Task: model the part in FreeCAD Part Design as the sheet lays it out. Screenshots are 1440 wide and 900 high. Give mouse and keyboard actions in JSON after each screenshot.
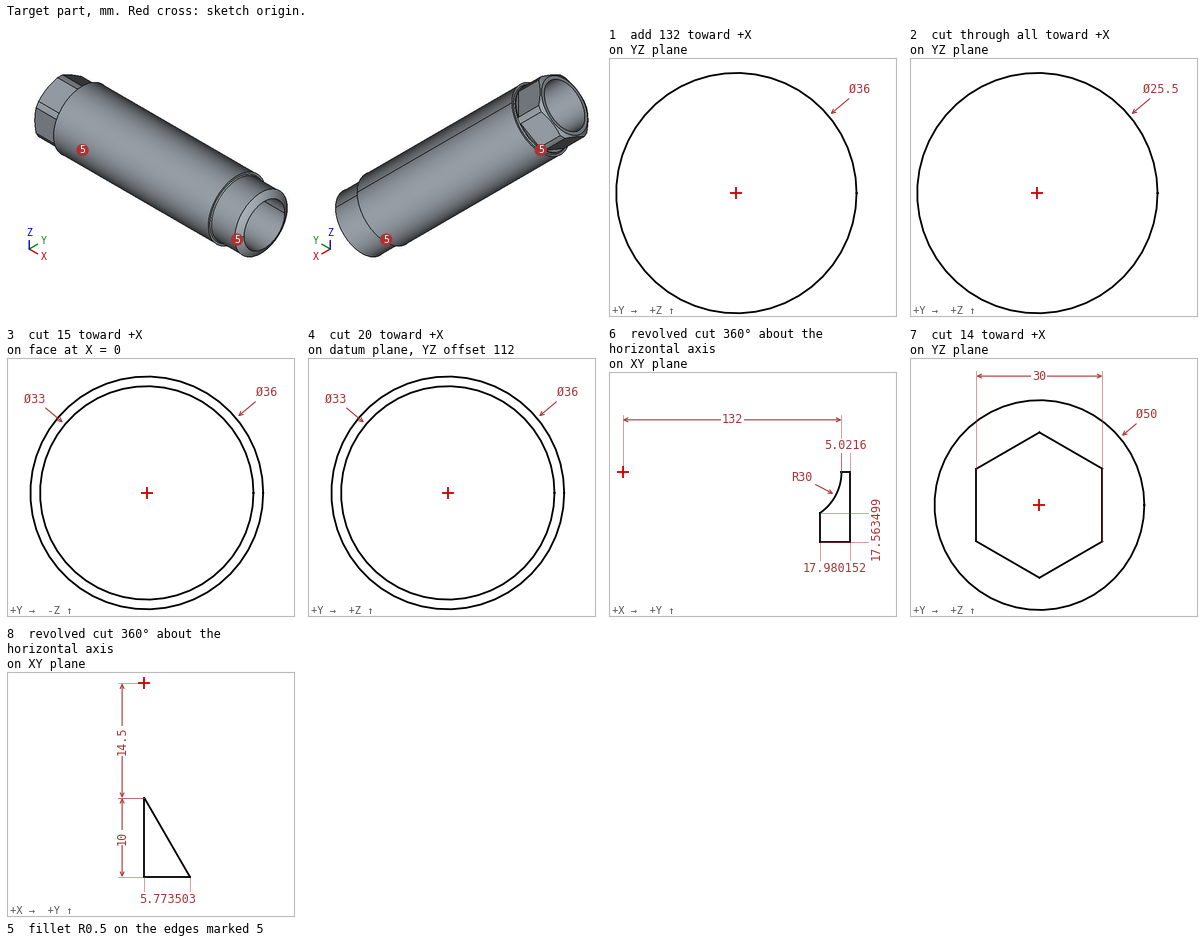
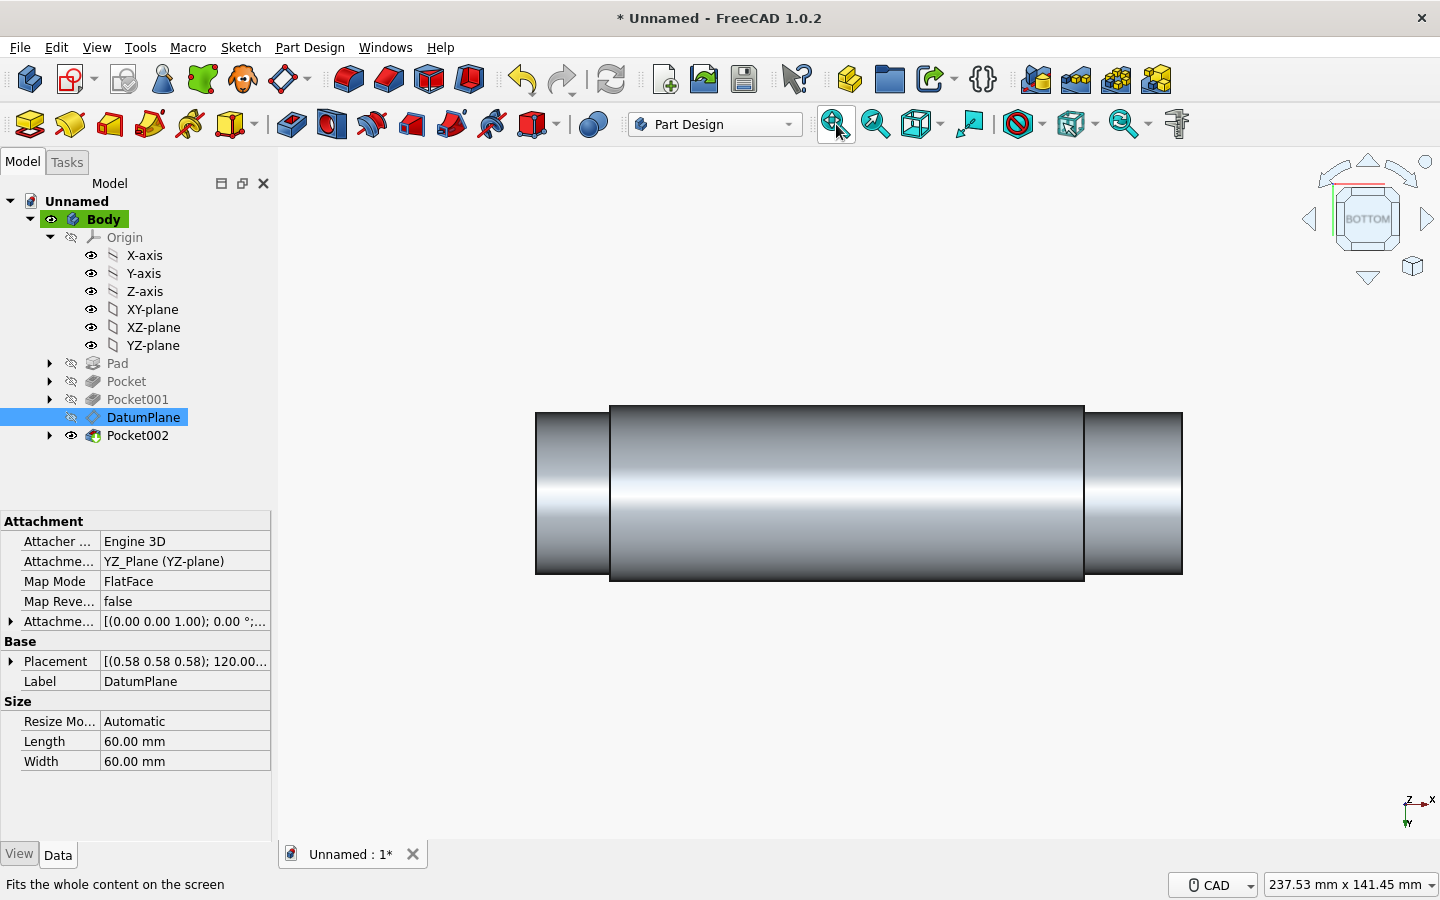
{"action": "key", "text": "4"}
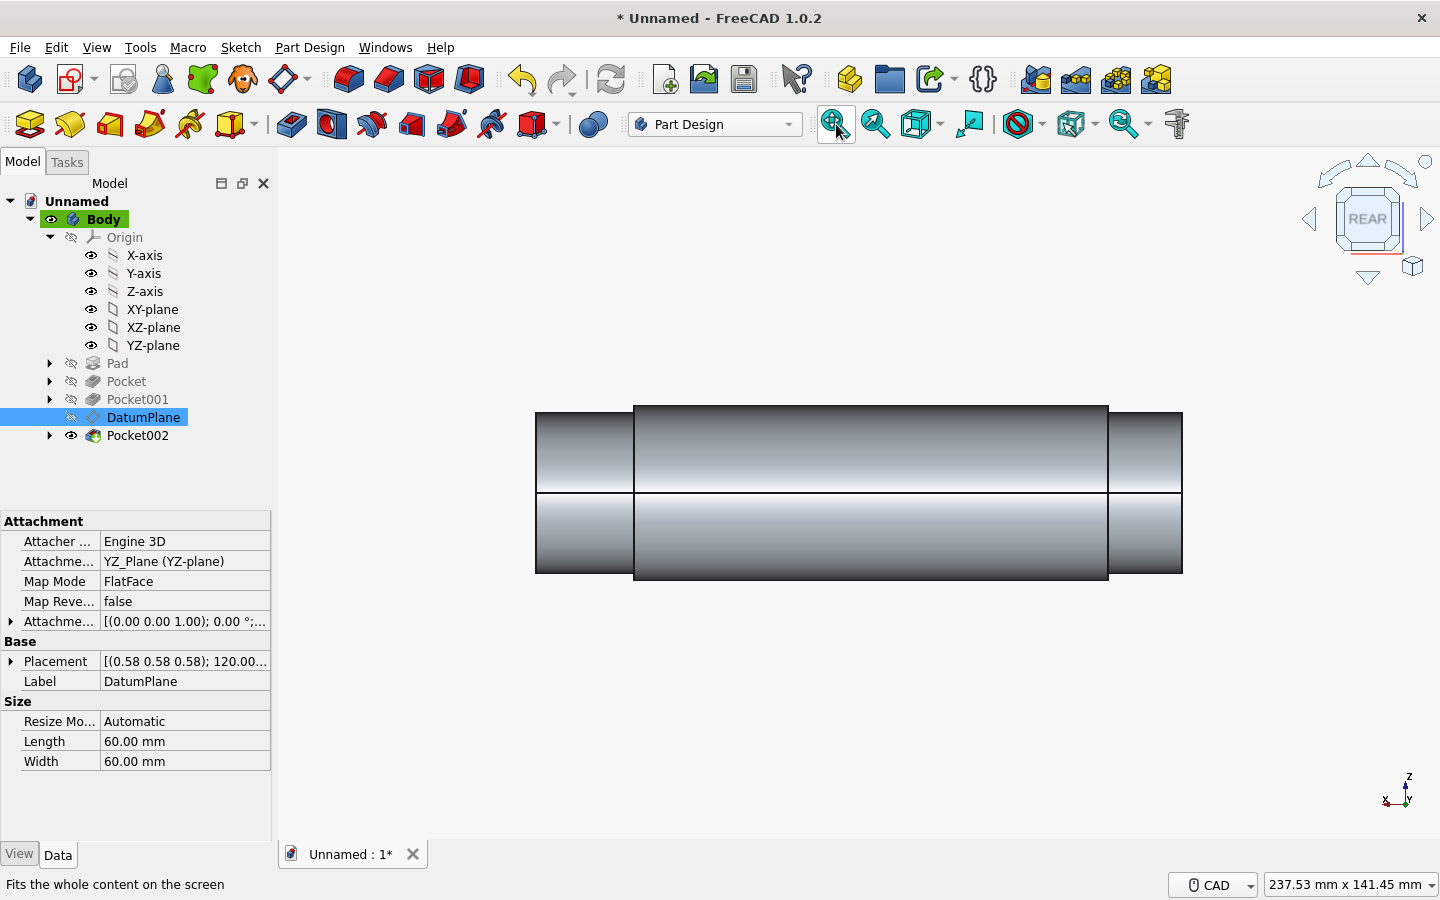
{"action": "key", "text": "6"}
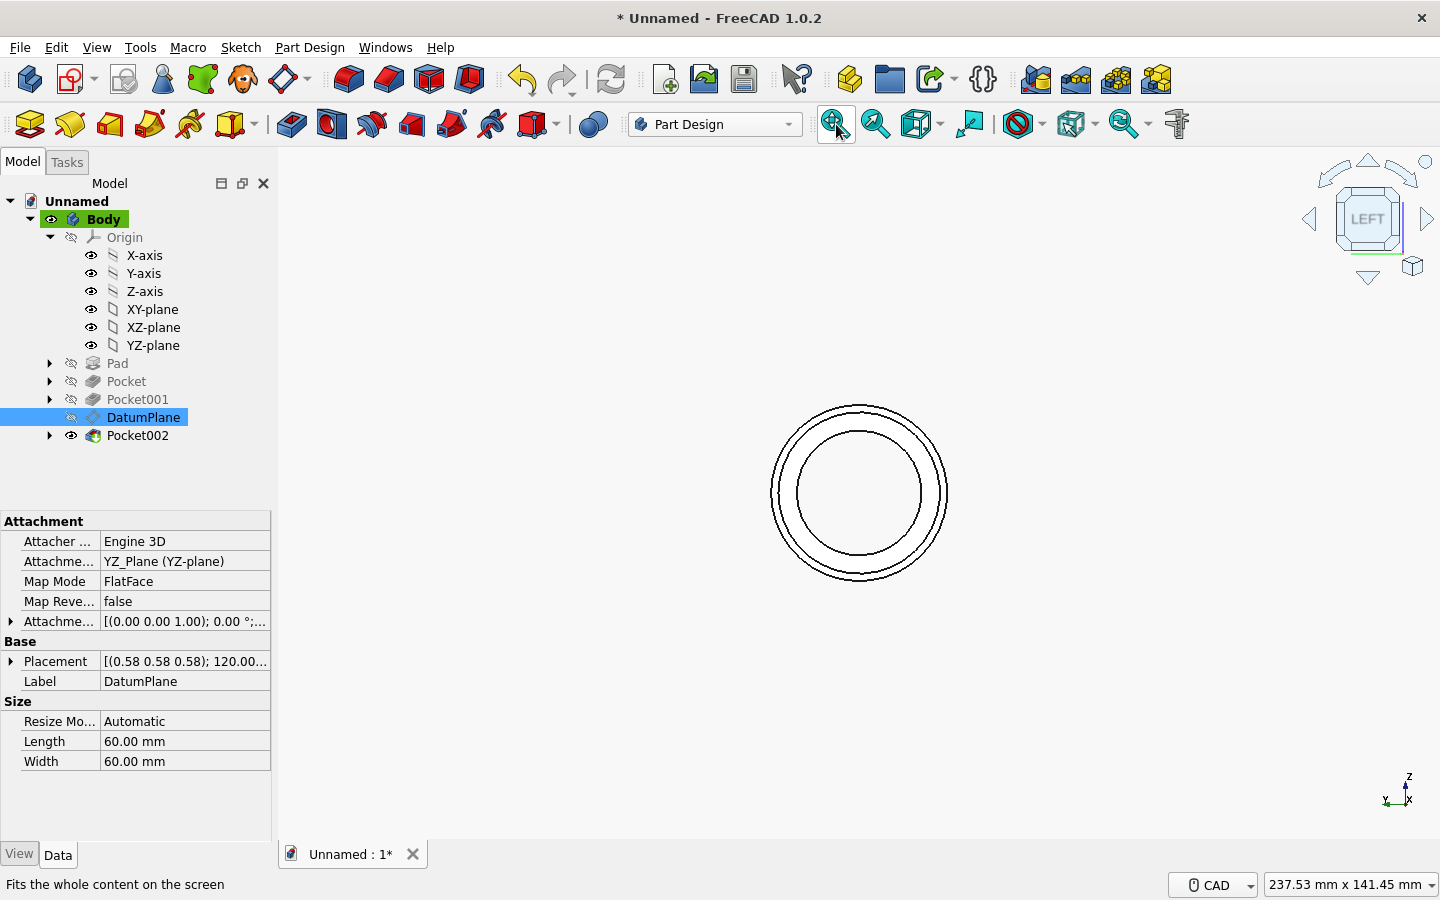
{"action": "left_click", "coordinate": [836, 124]}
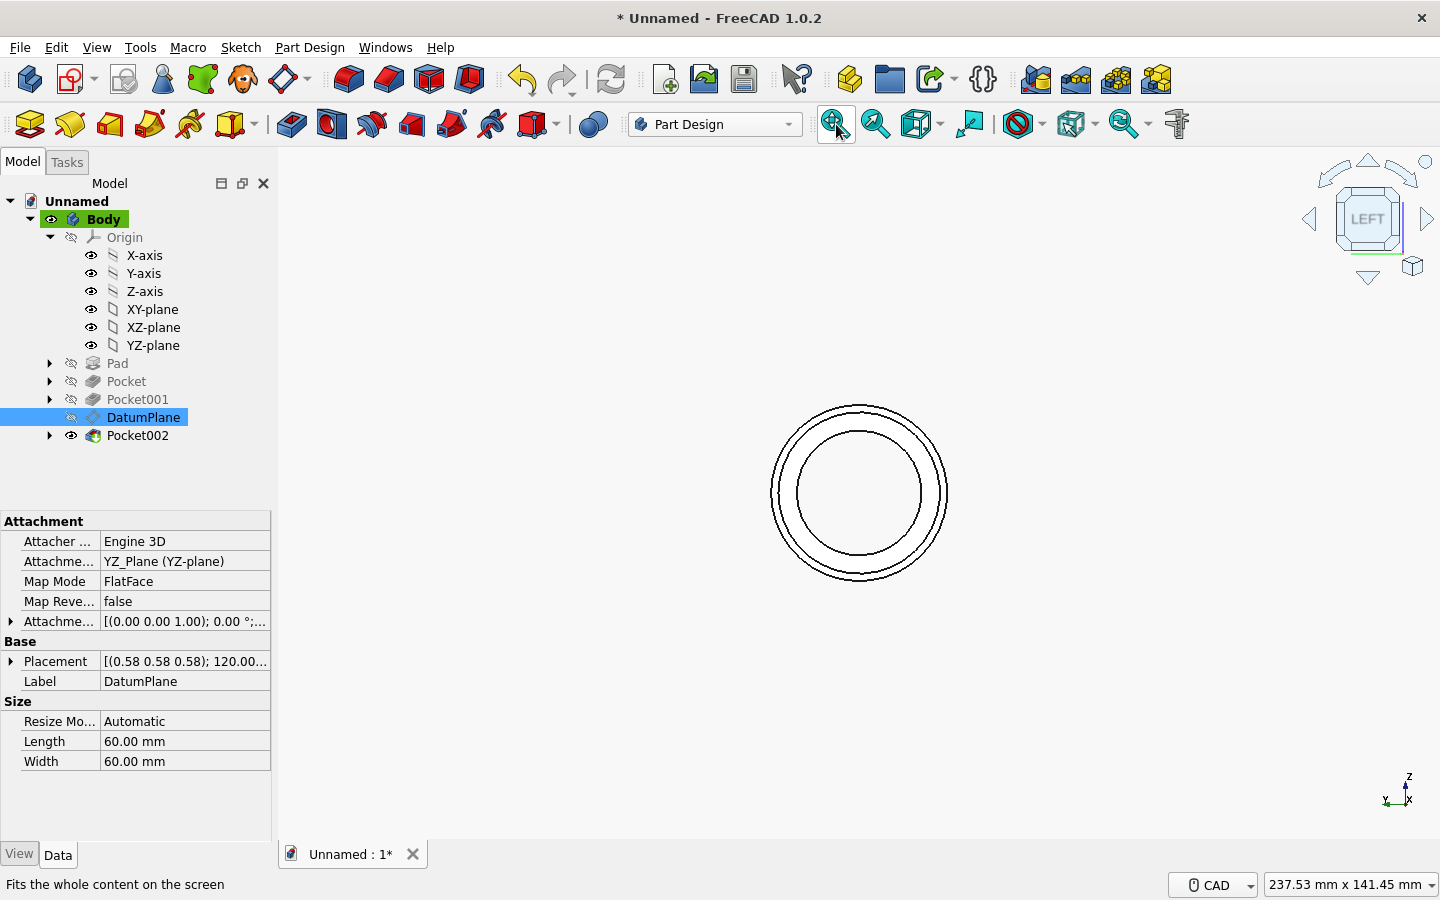
{"action": "key", "text": "v 3"}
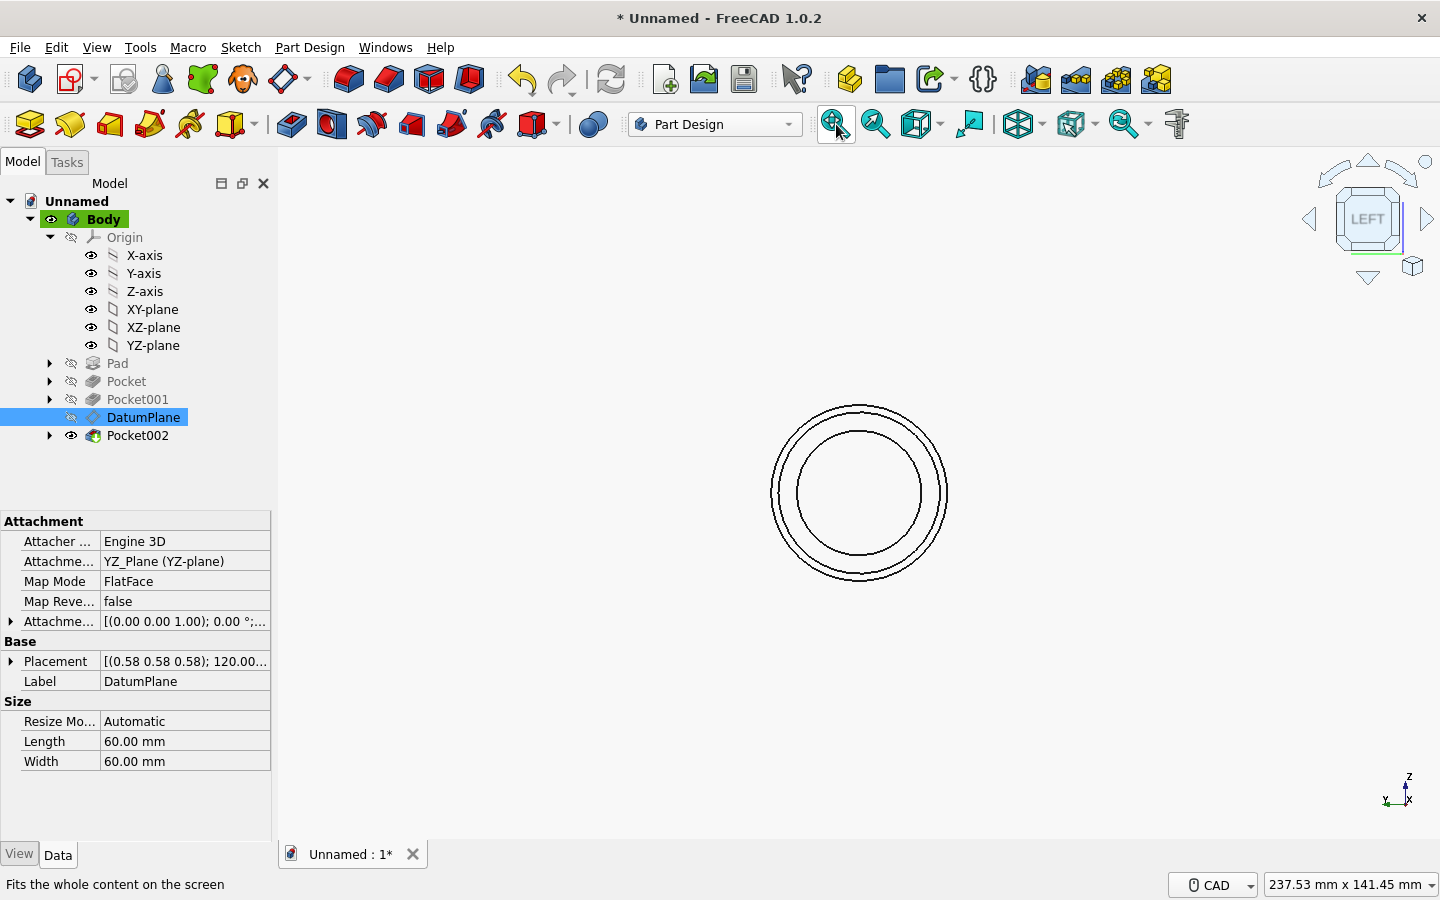
{"action": "key", "text": "0"}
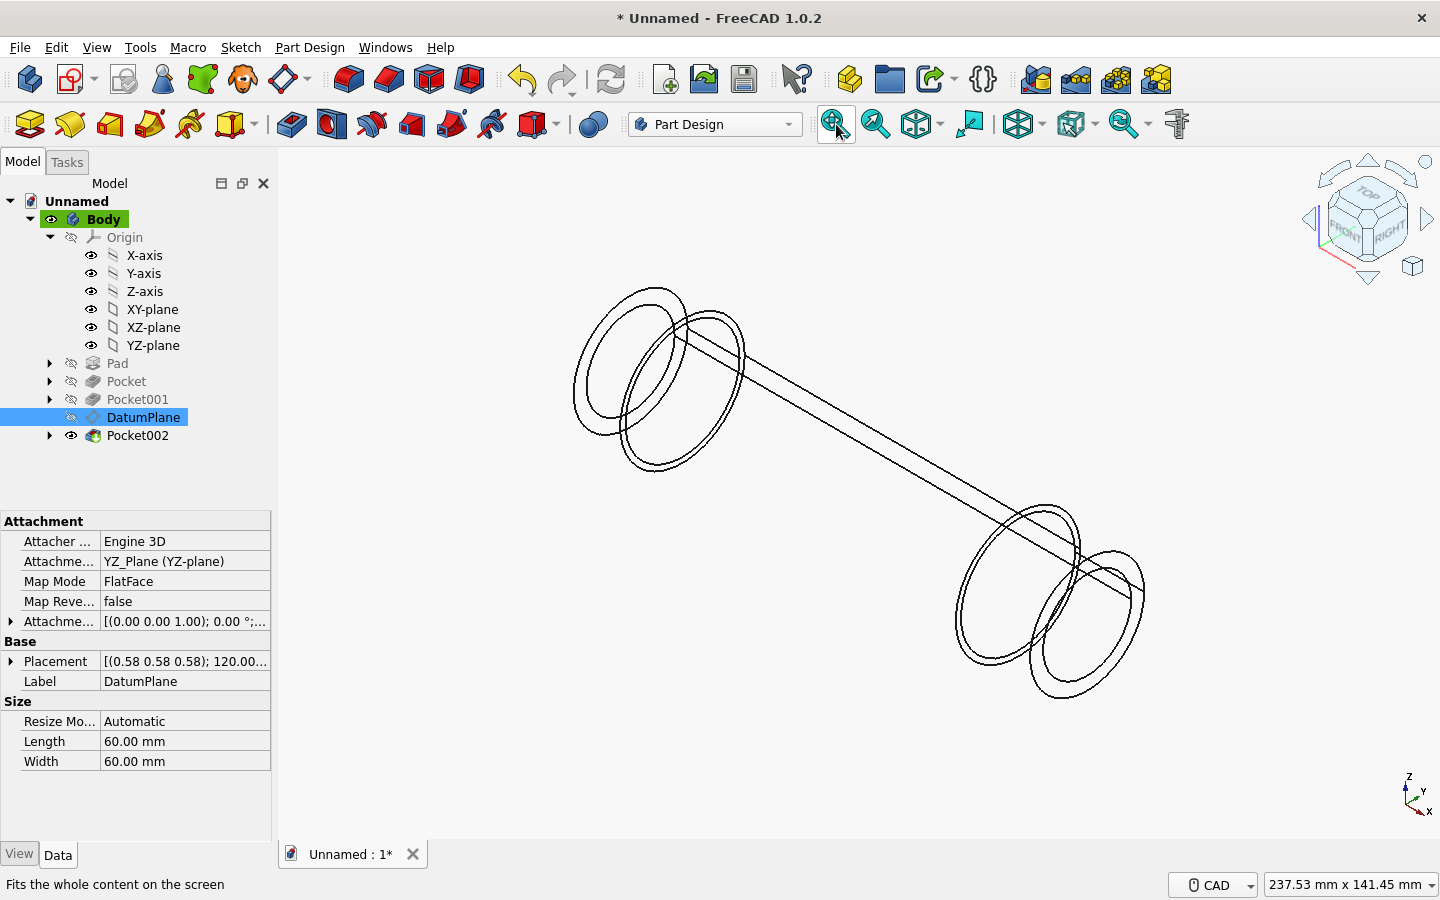
{"action": "left_click", "coordinate": [636, 456]}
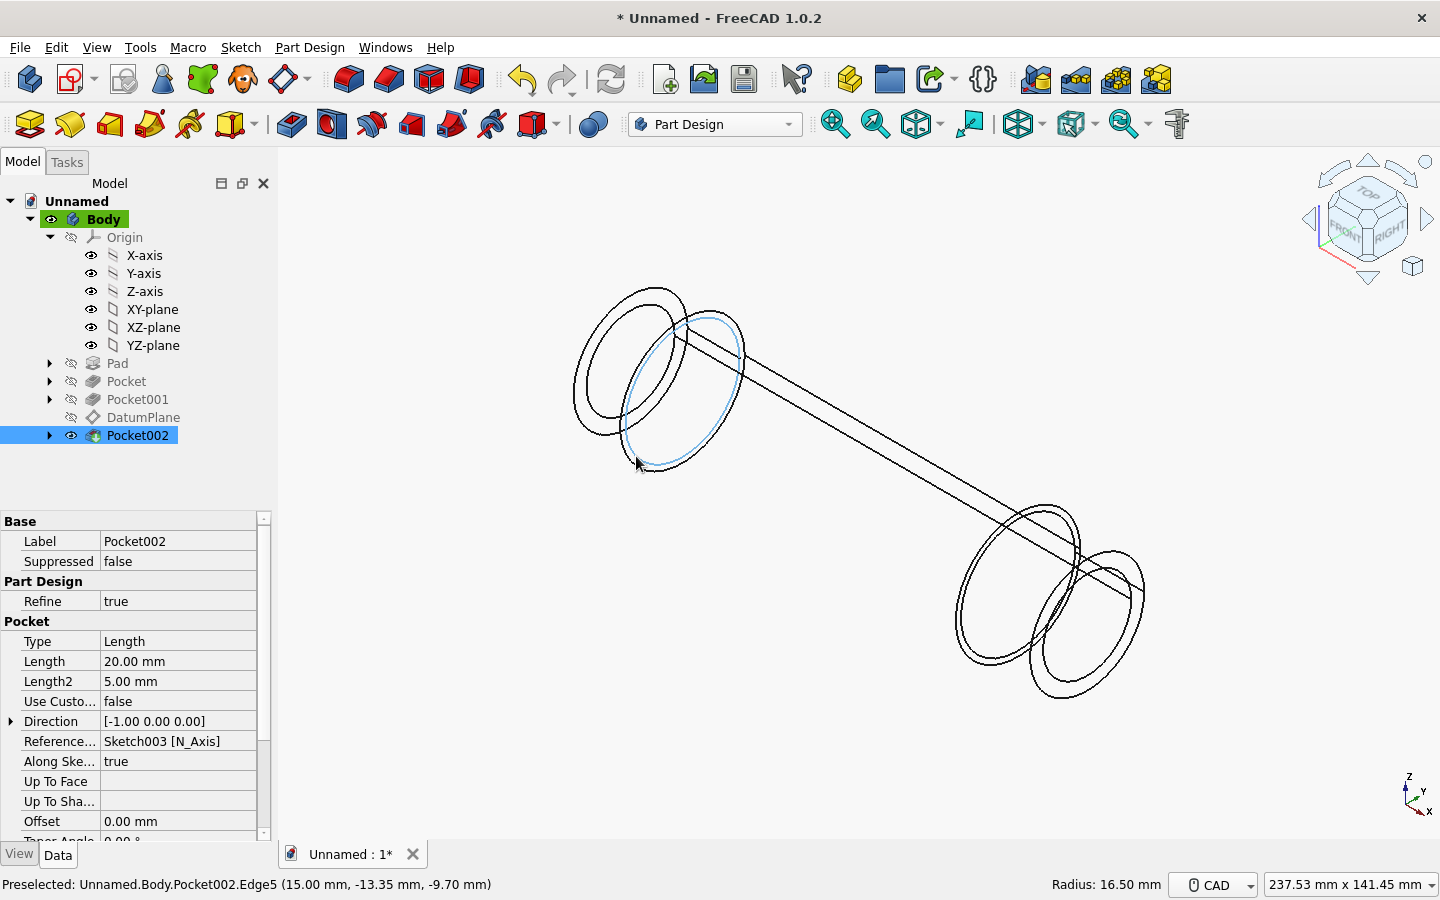
{"action": "left_click", "coordinate": [972, 649], "text": "ctrl"}